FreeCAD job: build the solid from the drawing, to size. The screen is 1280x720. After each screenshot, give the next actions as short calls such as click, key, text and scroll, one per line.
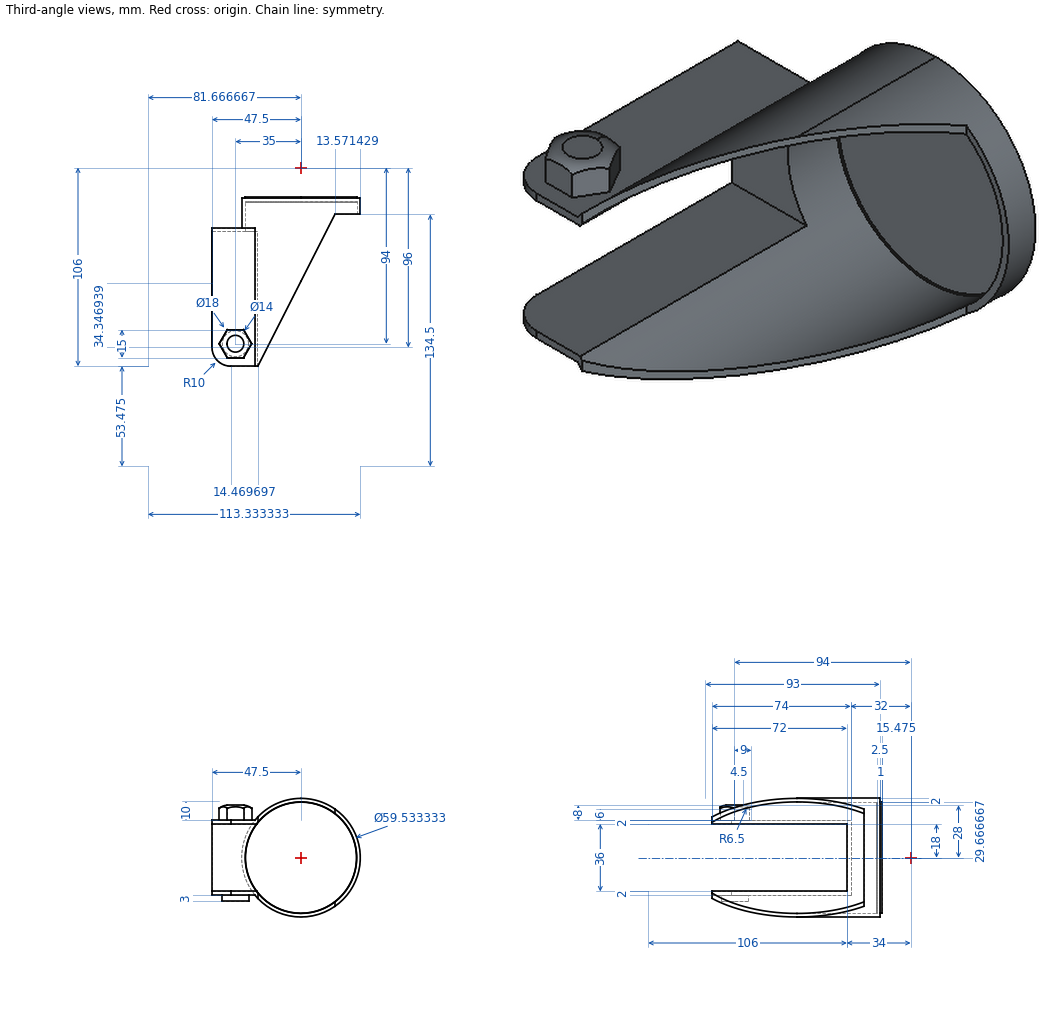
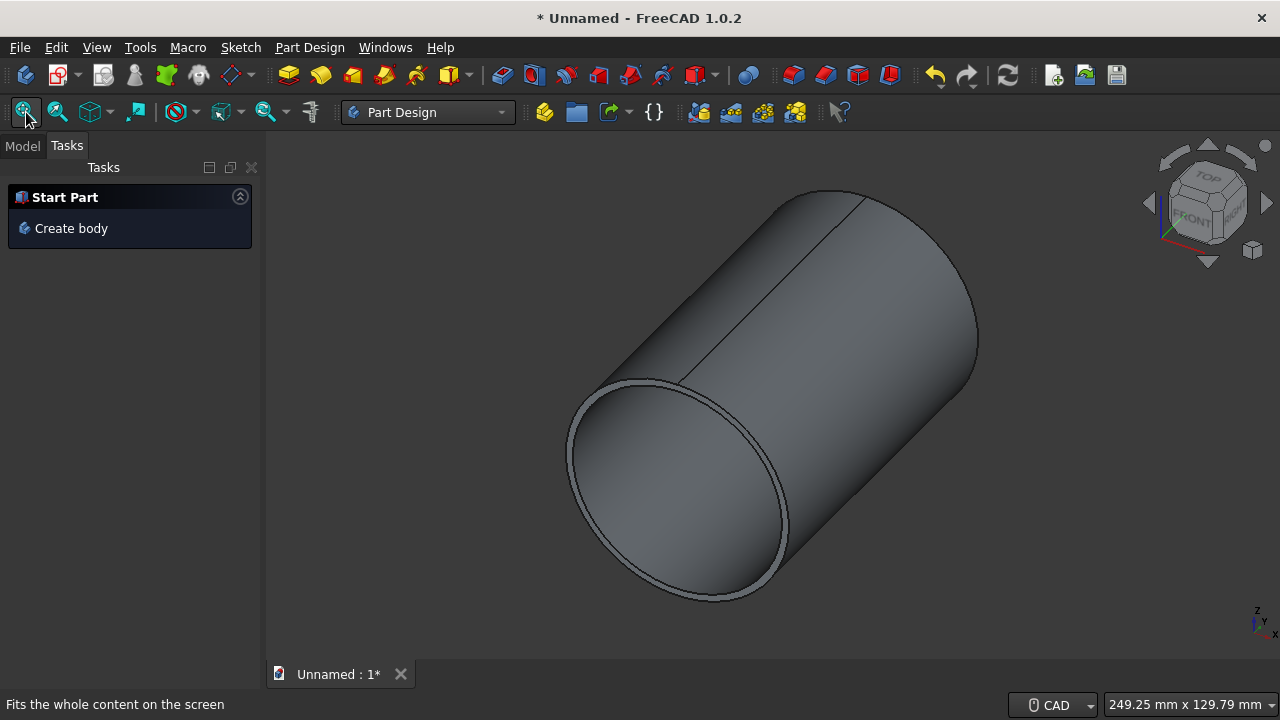
click(58, 76)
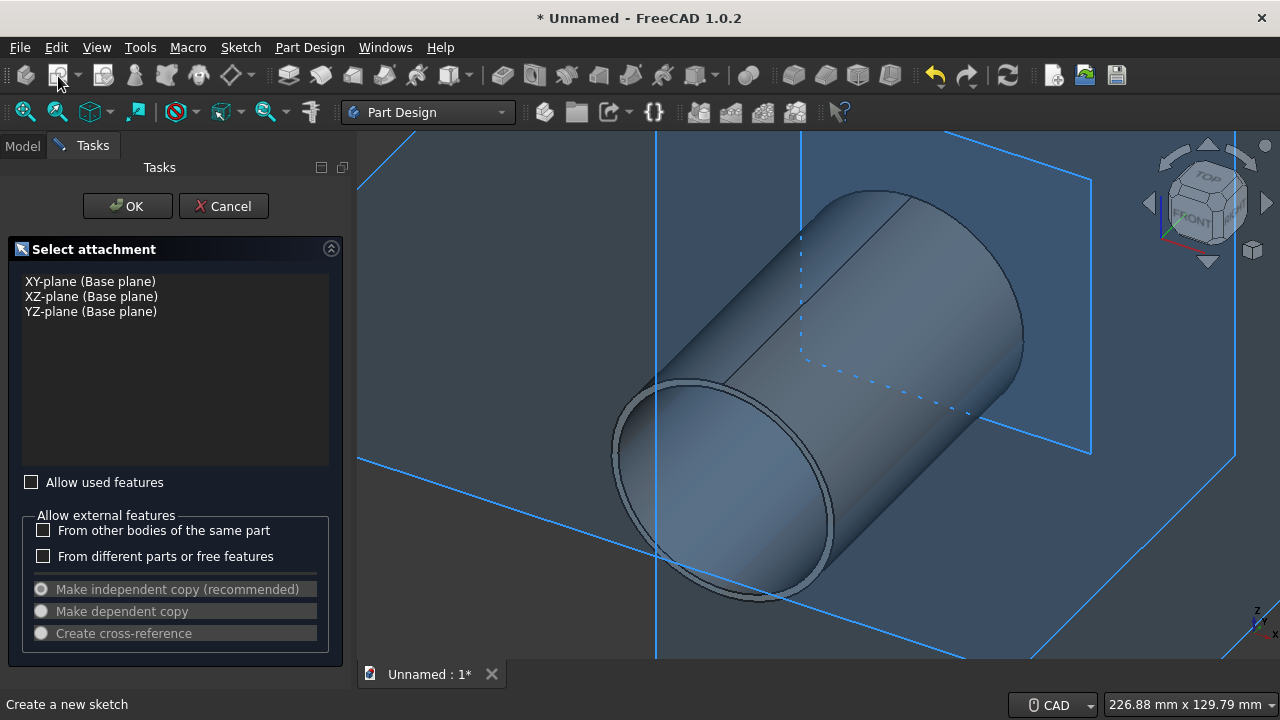
click(82, 312)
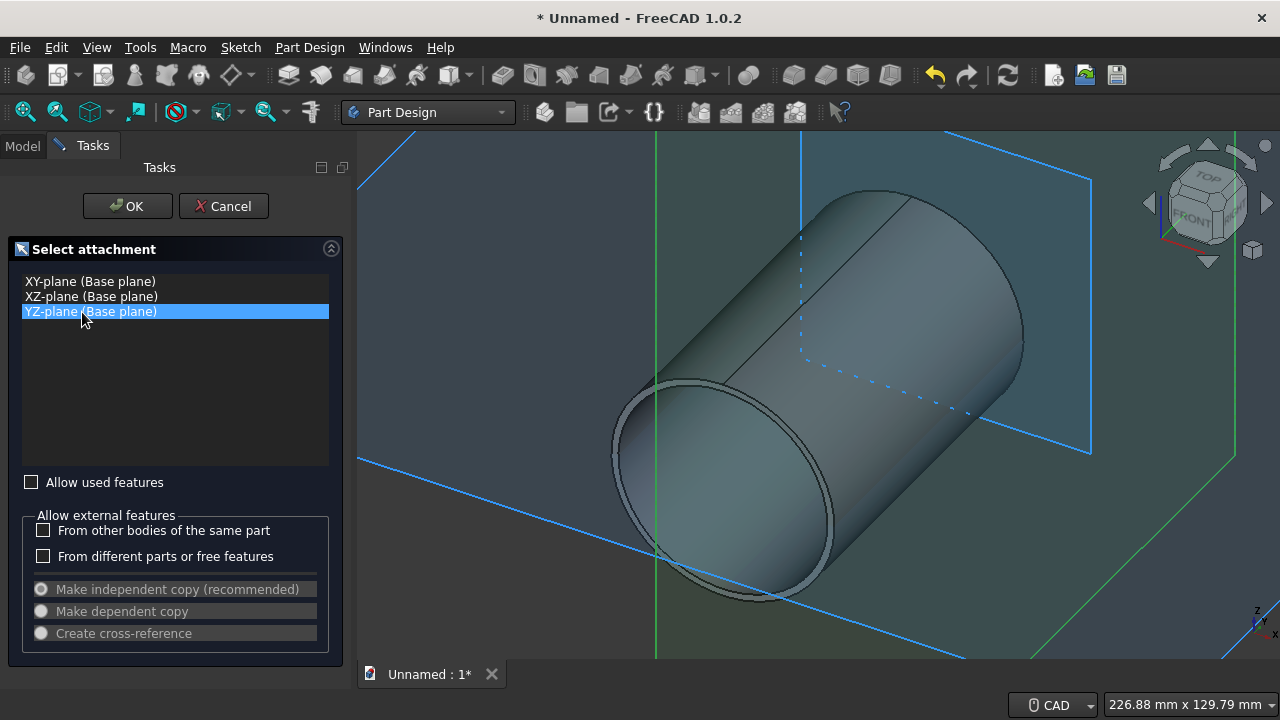
click(128, 206)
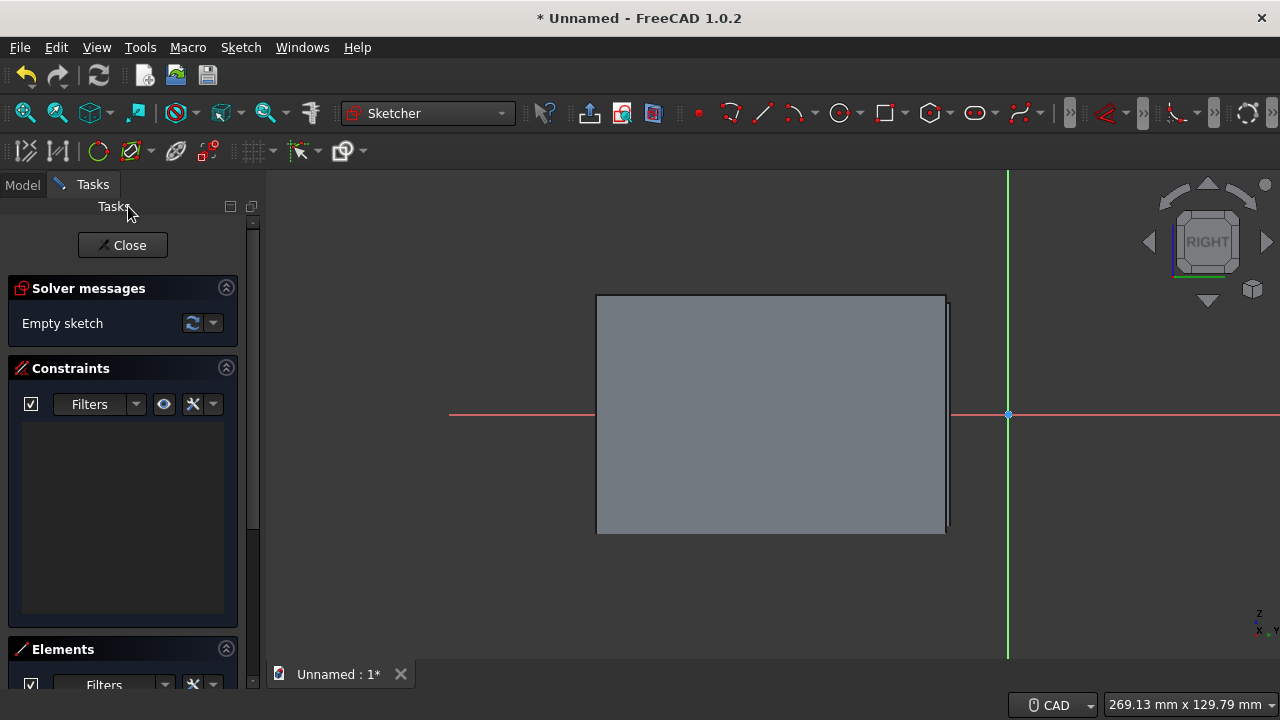
click(654, 114)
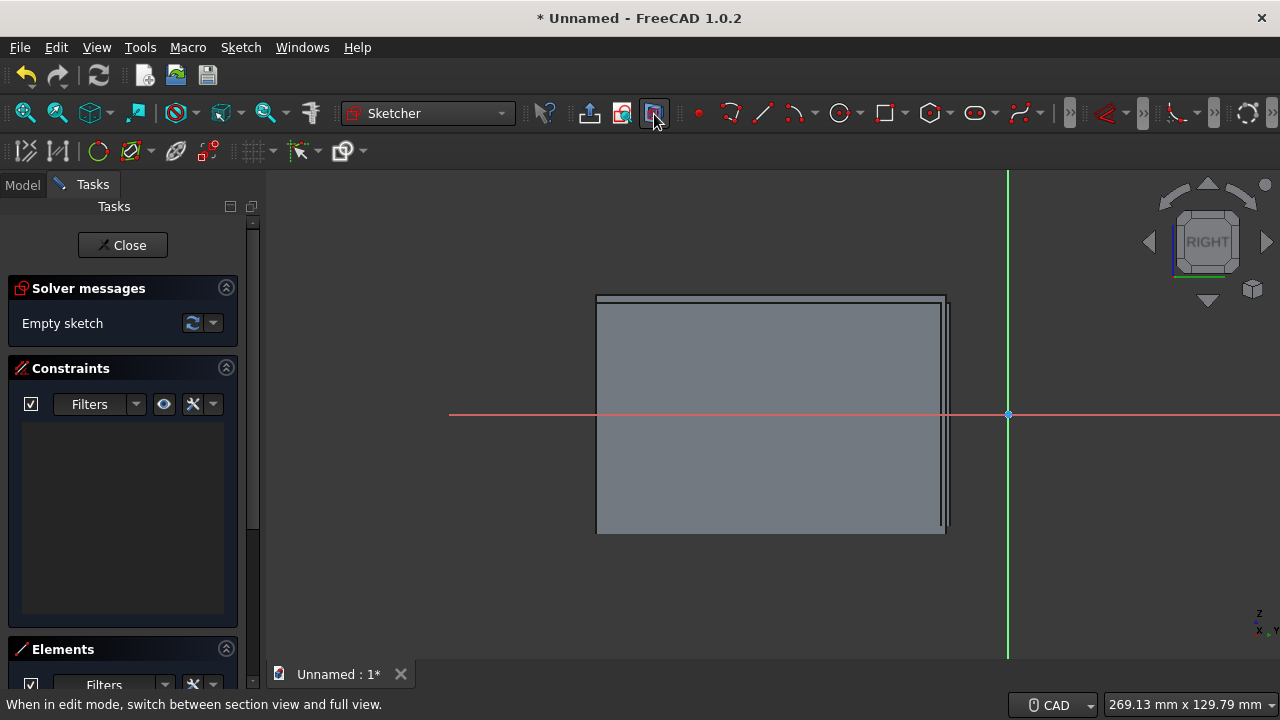
key(g)
key(r)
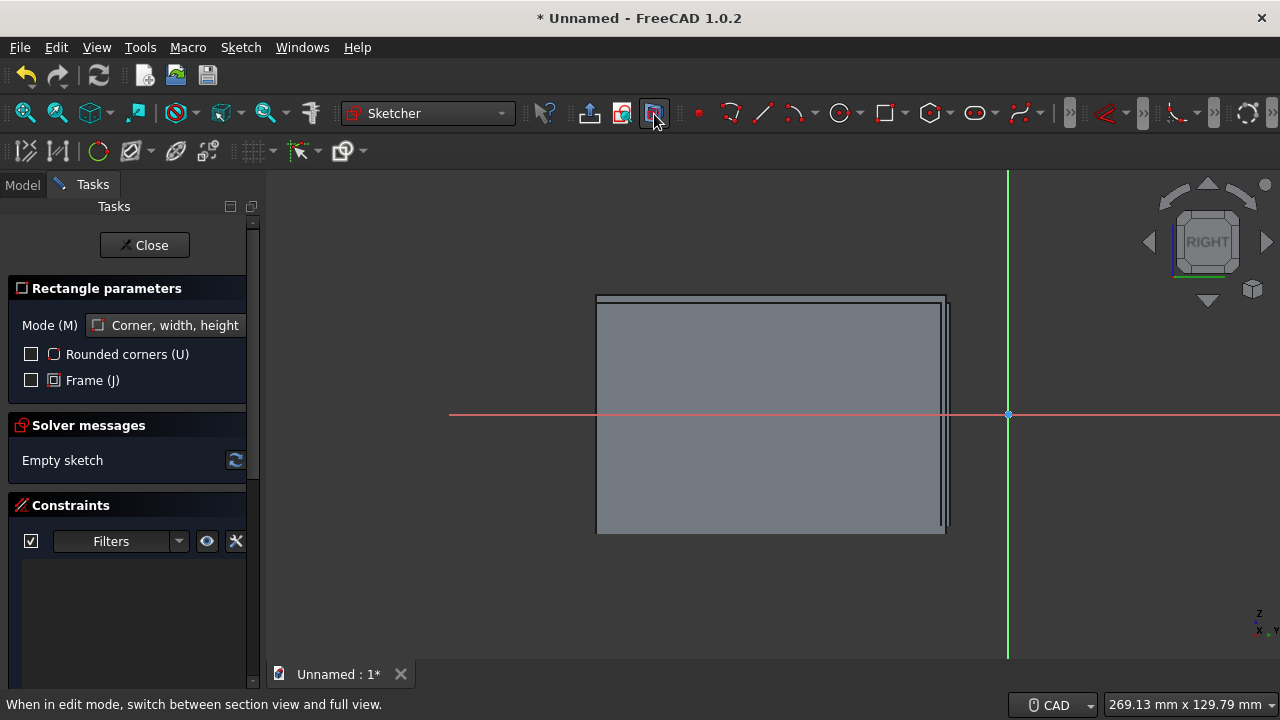
click(481, 347)
click(880, 482)
key(Escape)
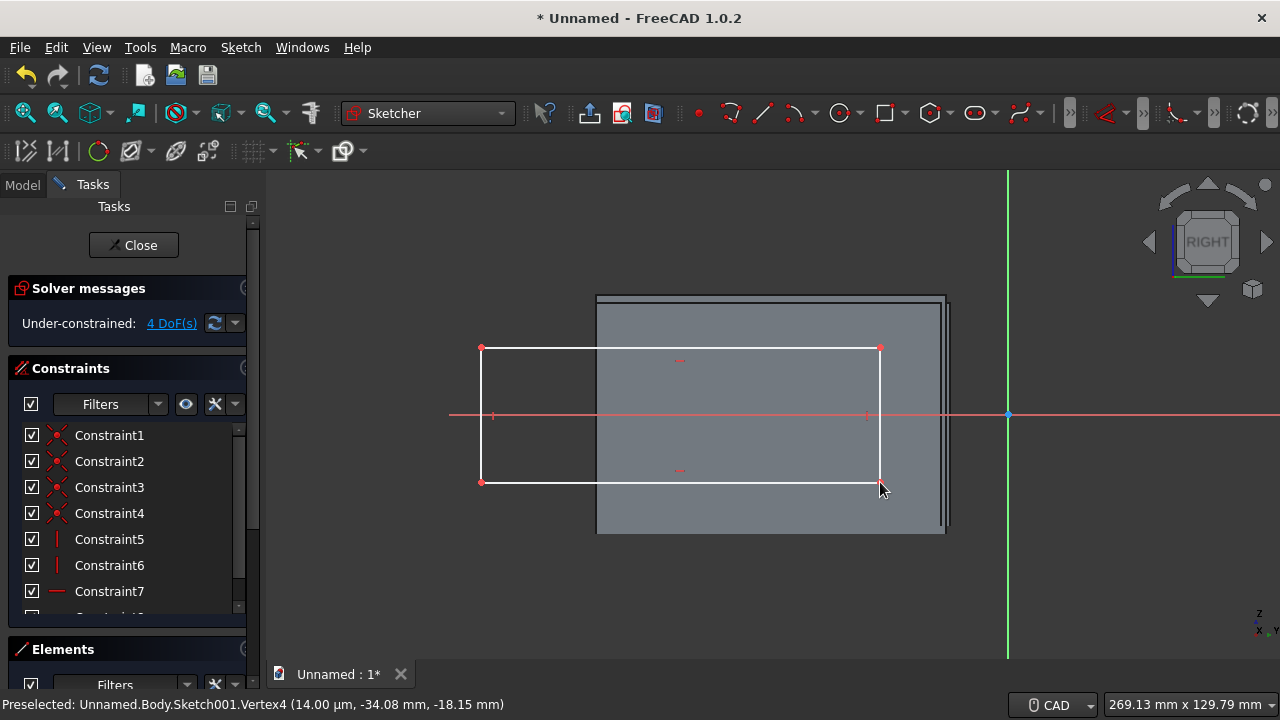
key(d)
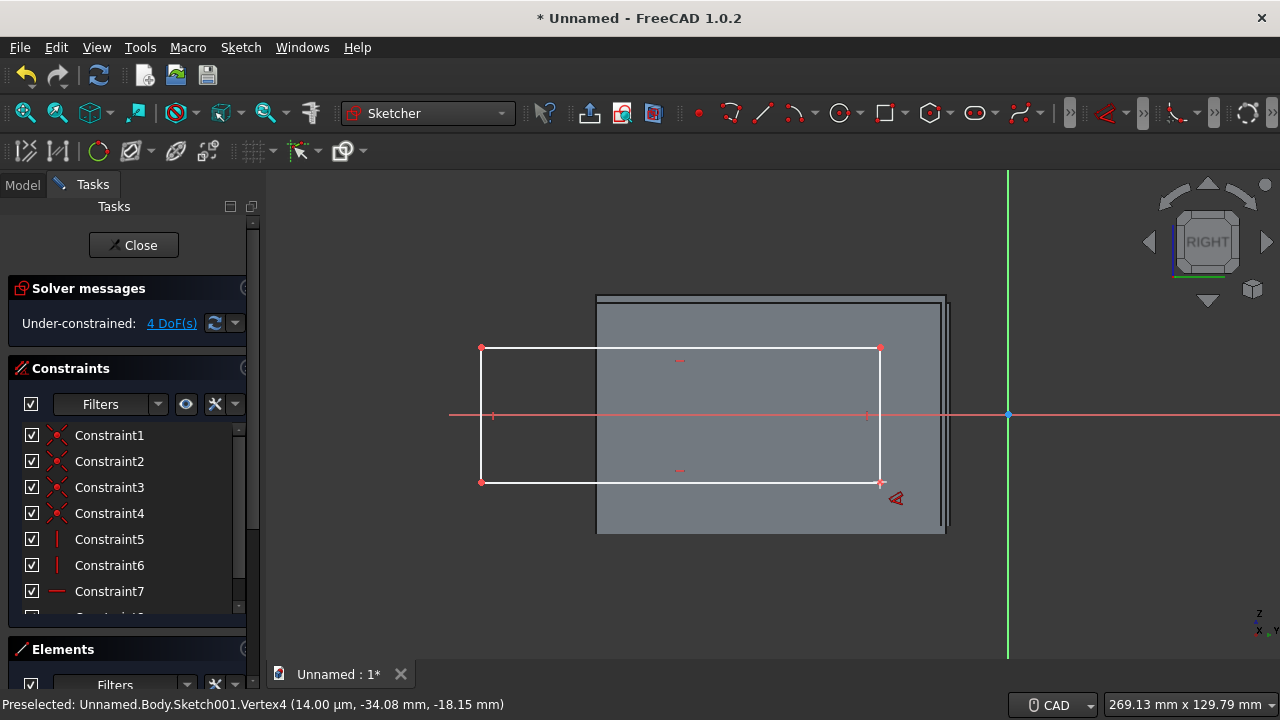
click(481, 389)
click(447, 384)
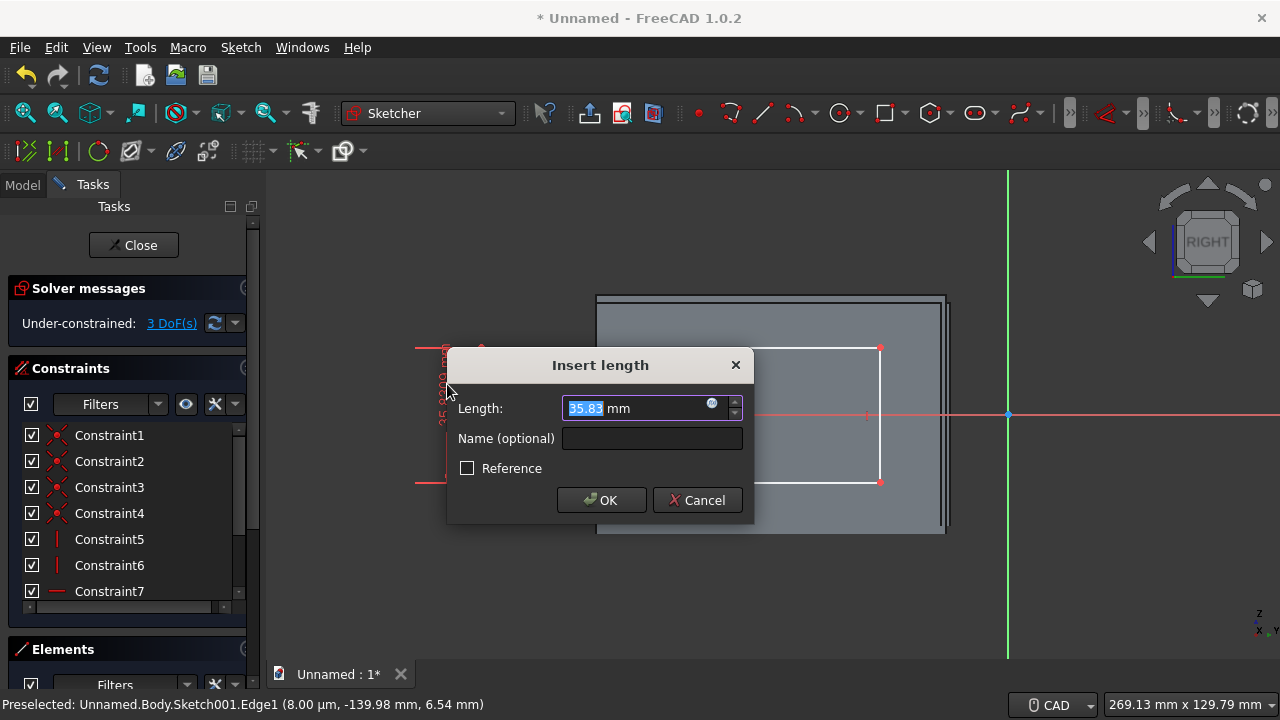
text(36)
key(Return)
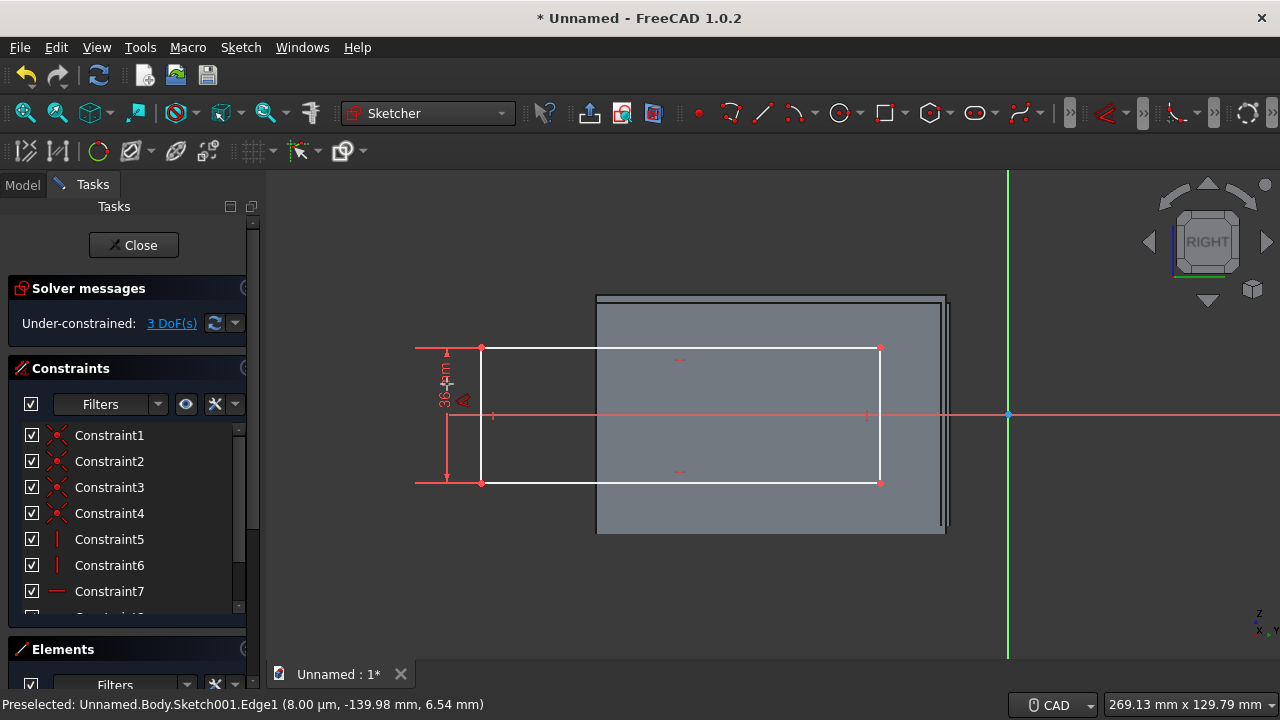
click(601, 483)
click(681, 517)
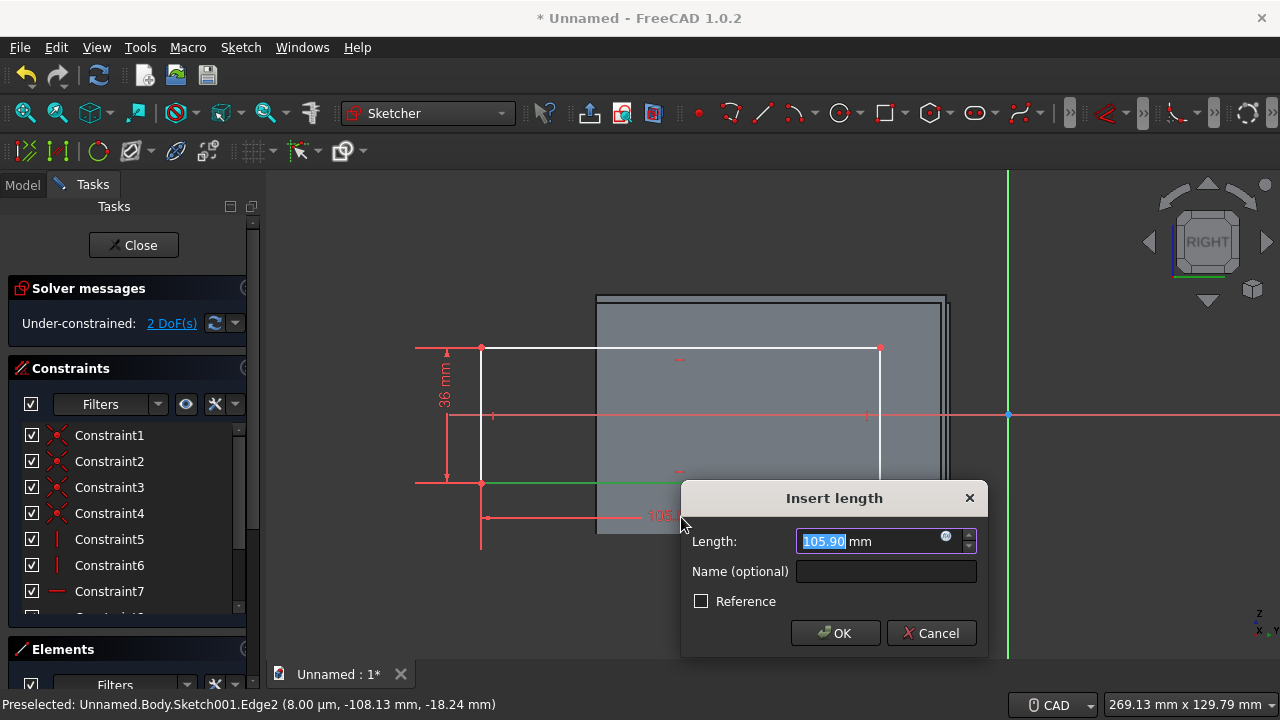
text(106)
key(Return)